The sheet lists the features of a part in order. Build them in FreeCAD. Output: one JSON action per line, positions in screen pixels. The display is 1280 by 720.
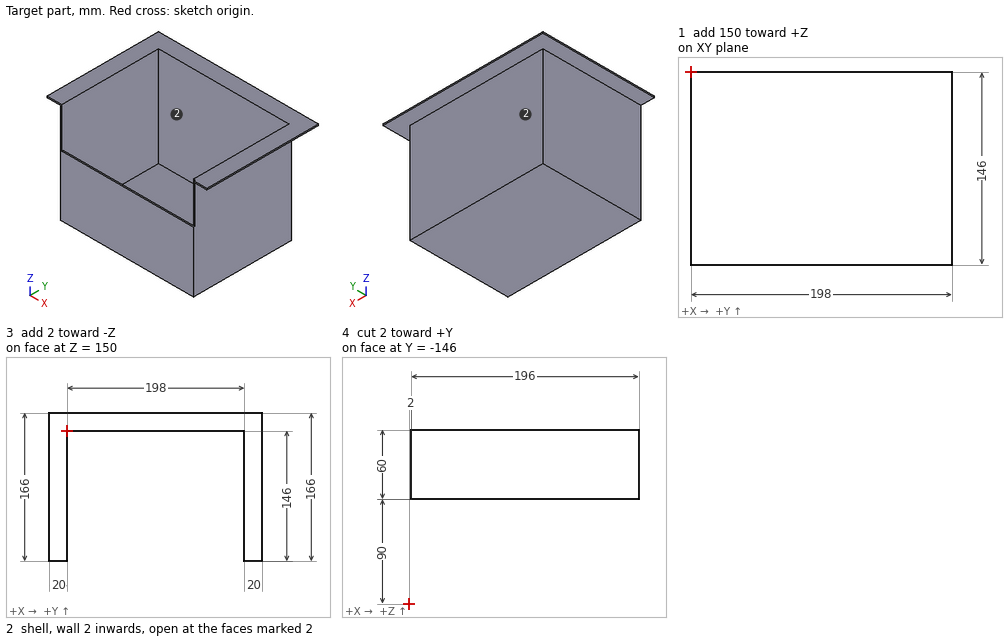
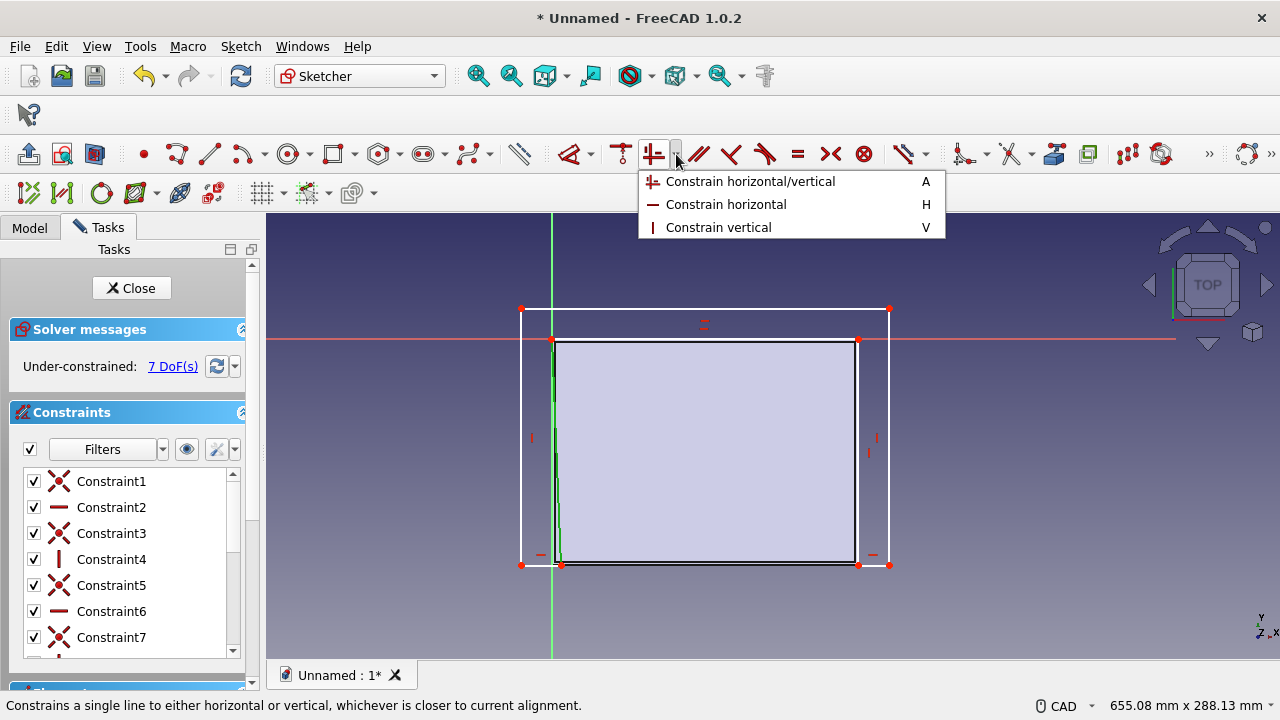
{"action": "left_click", "coordinate": [792, 228]}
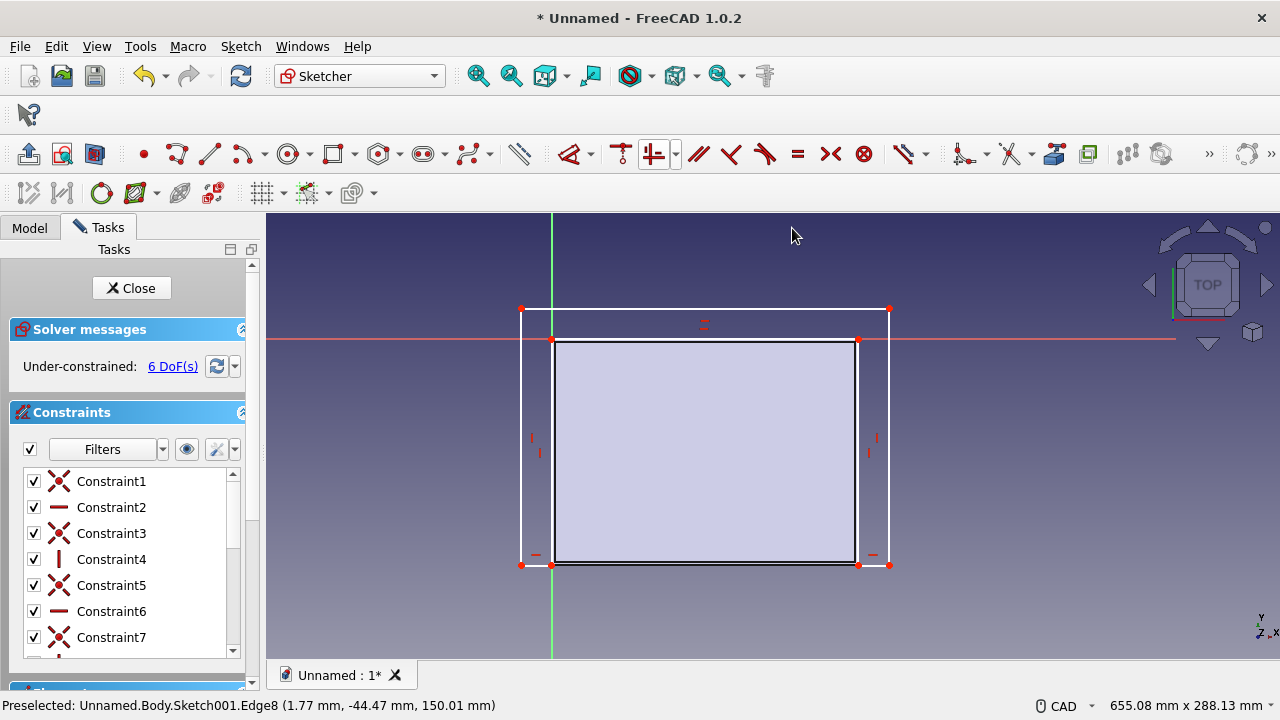
{"action": "left_click", "coordinate": [568, 154]}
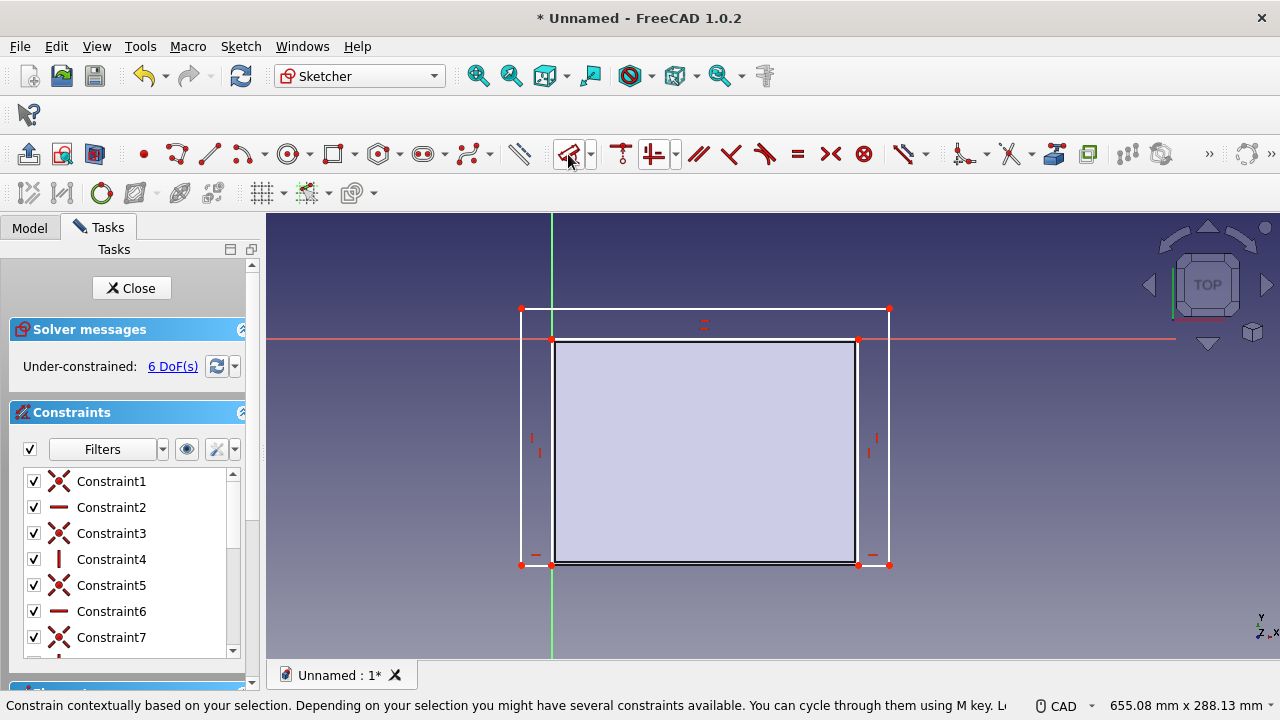
{"action": "scroll", "coordinate": [867, 566], "scroll_direction": "up", "scroll_amount": 2}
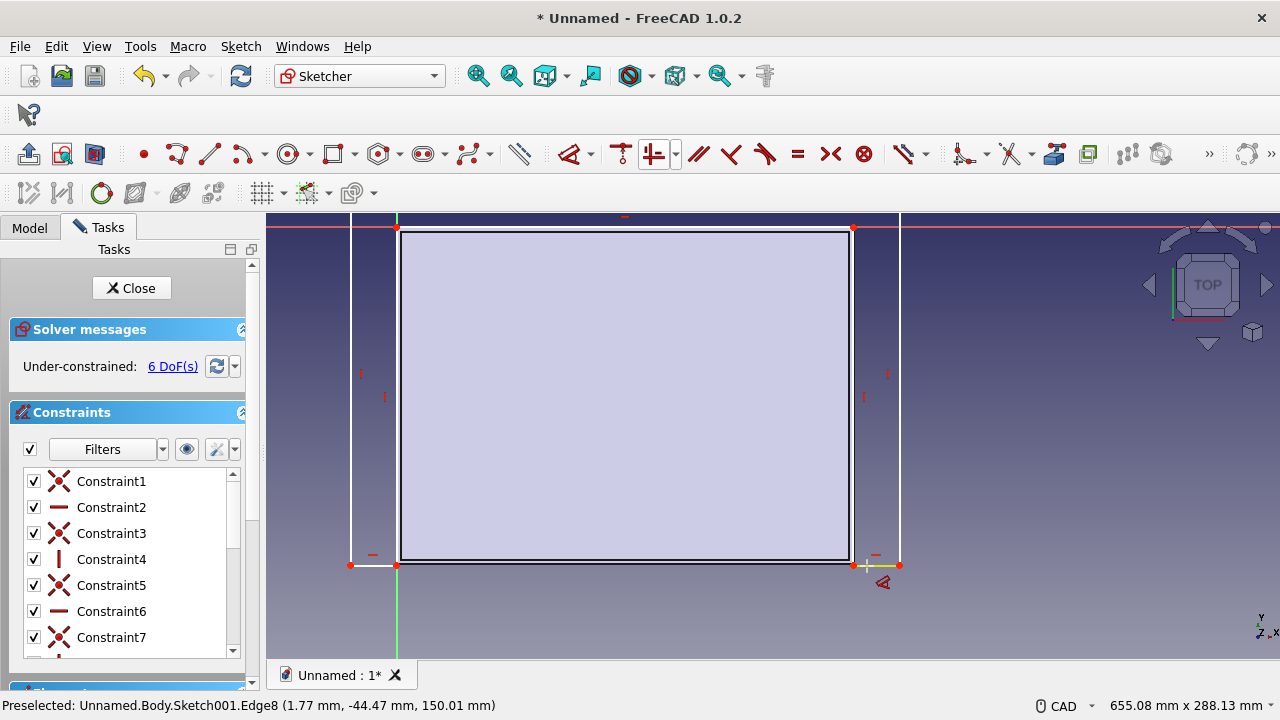
{"action": "left_click", "coordinate": [867, 566]}
{"action": "left_click", "coordinate": [876, 600]}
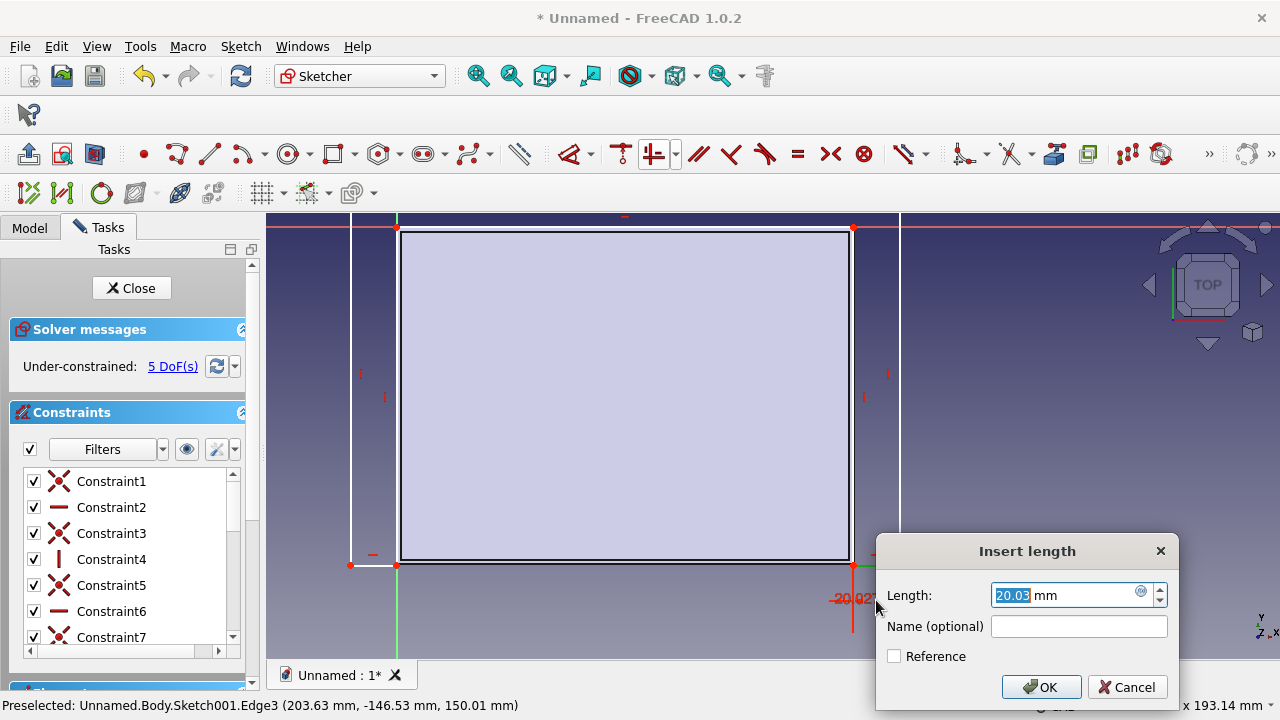
{"action": "type", "text": "20"}
{"action": "key", "text": "Return"}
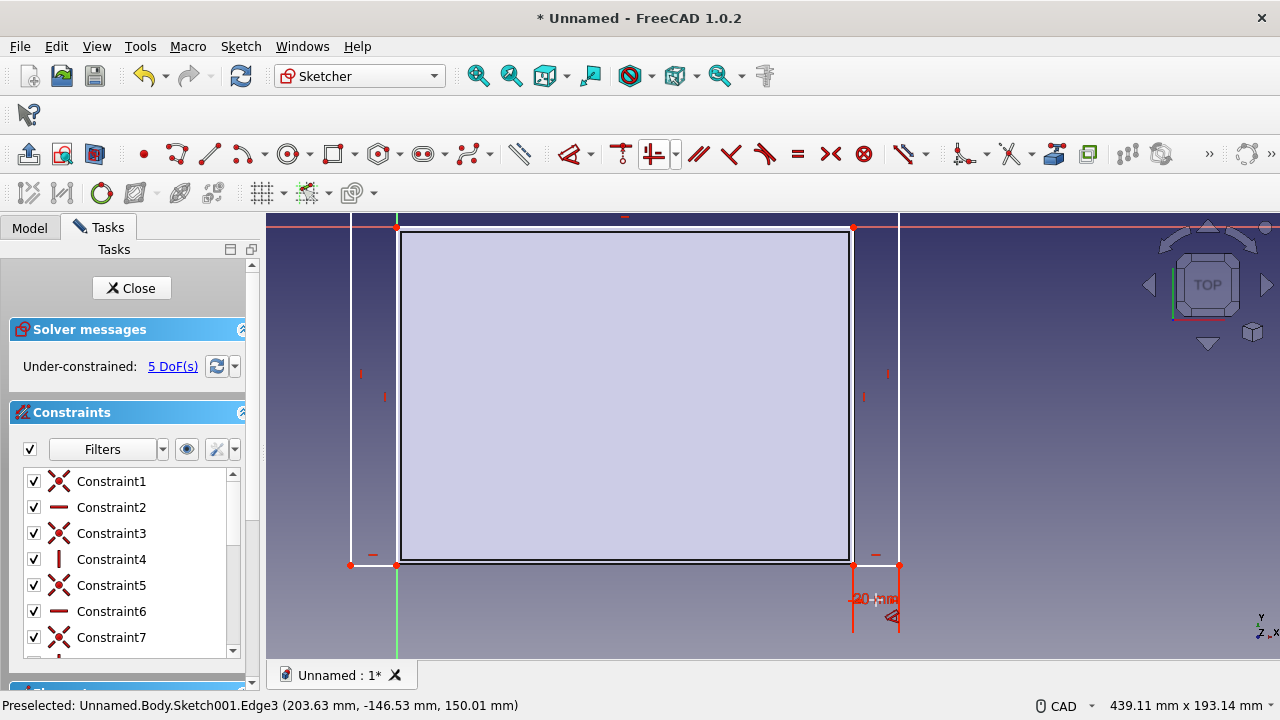
{"action": "left_click", "coordinate": [364, 566]}
{"action": "left_click", "coordinate": [374, 600]}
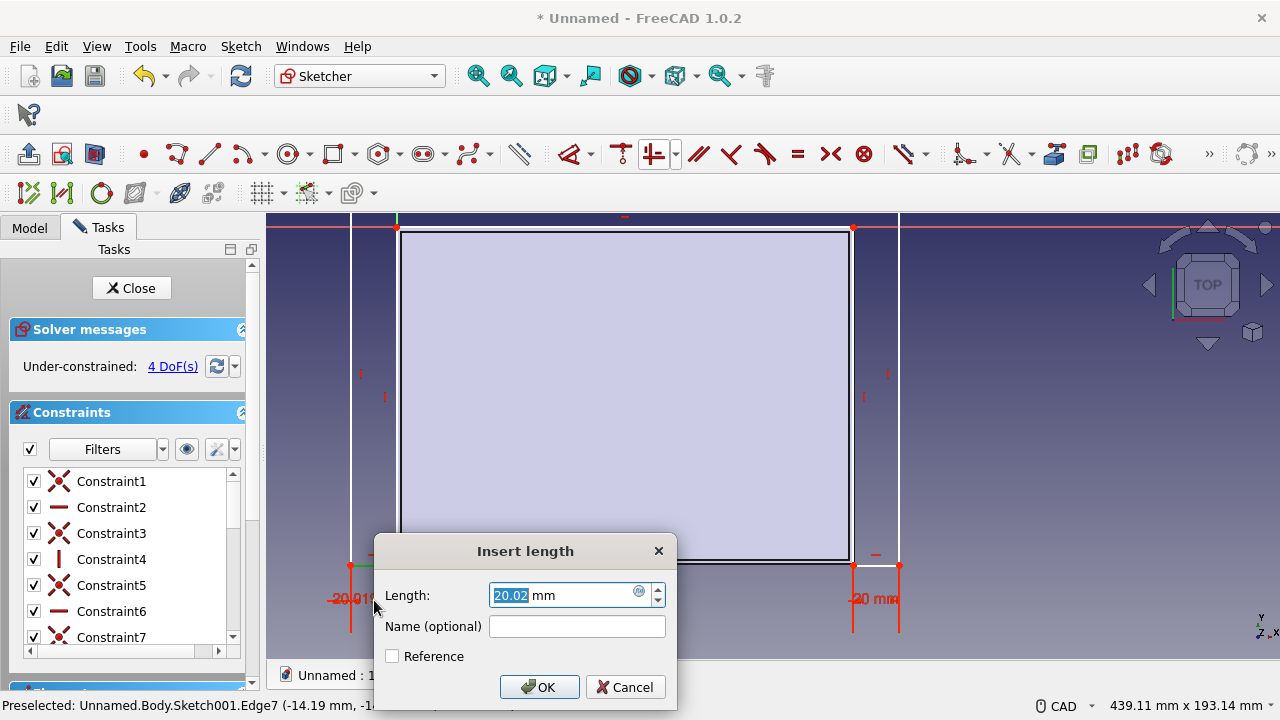
{"action": "type", "text": "20"}
{"action": "key", "text": "Return"}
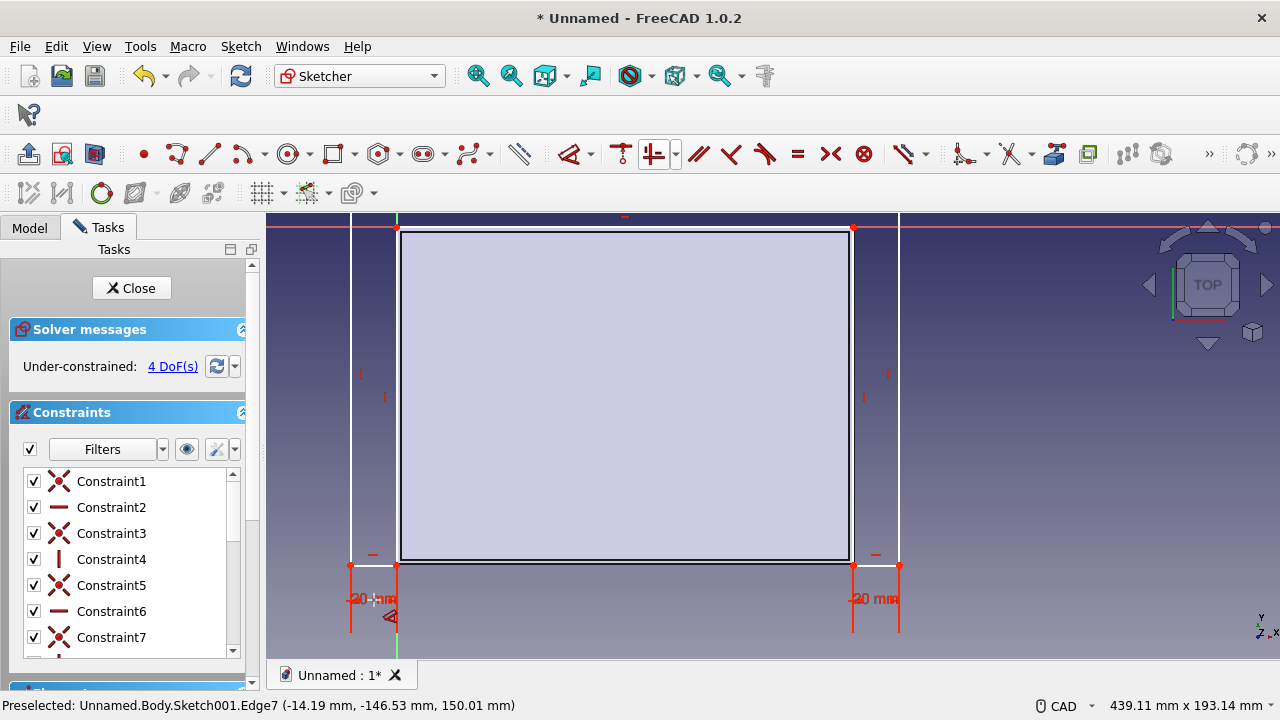
{"action": "scroll", "coordinate": [865, 565], "scroll_direction": "down", "scroll_amount": 2}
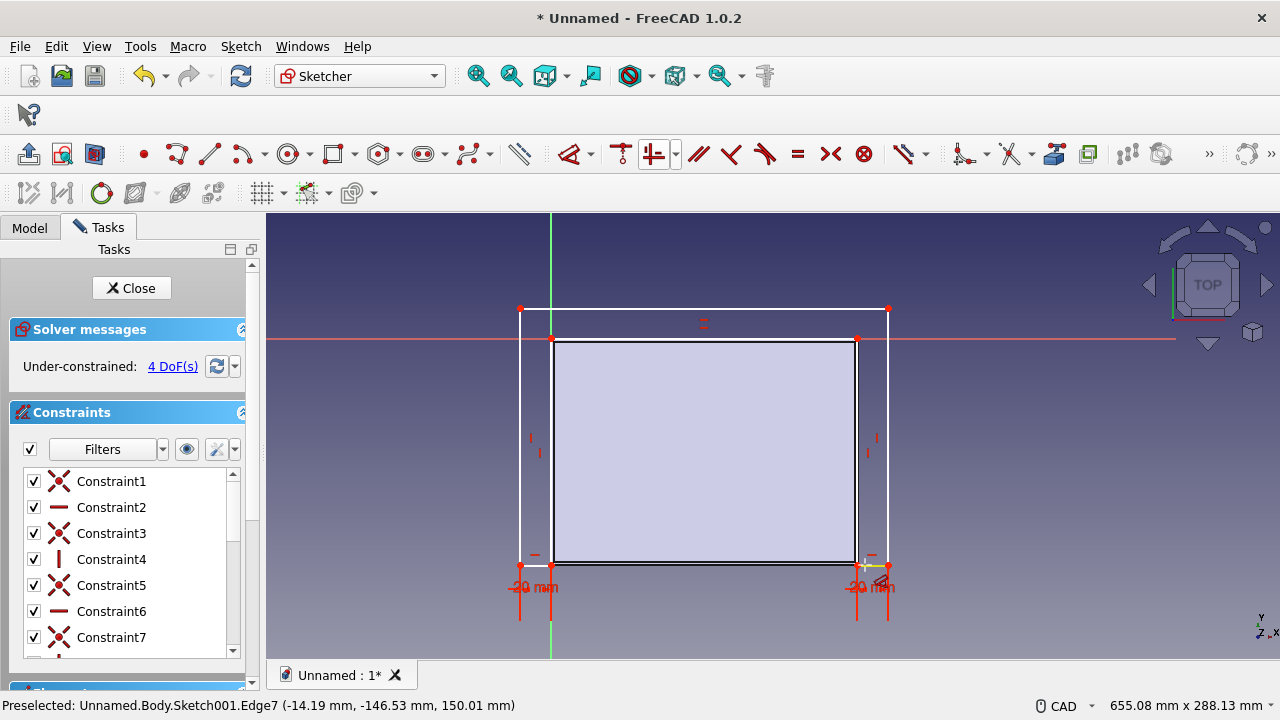
{"action": "left_click", "coordinate": [643, 339]}
{"action": "left_click", "coordinate": [704, 373]}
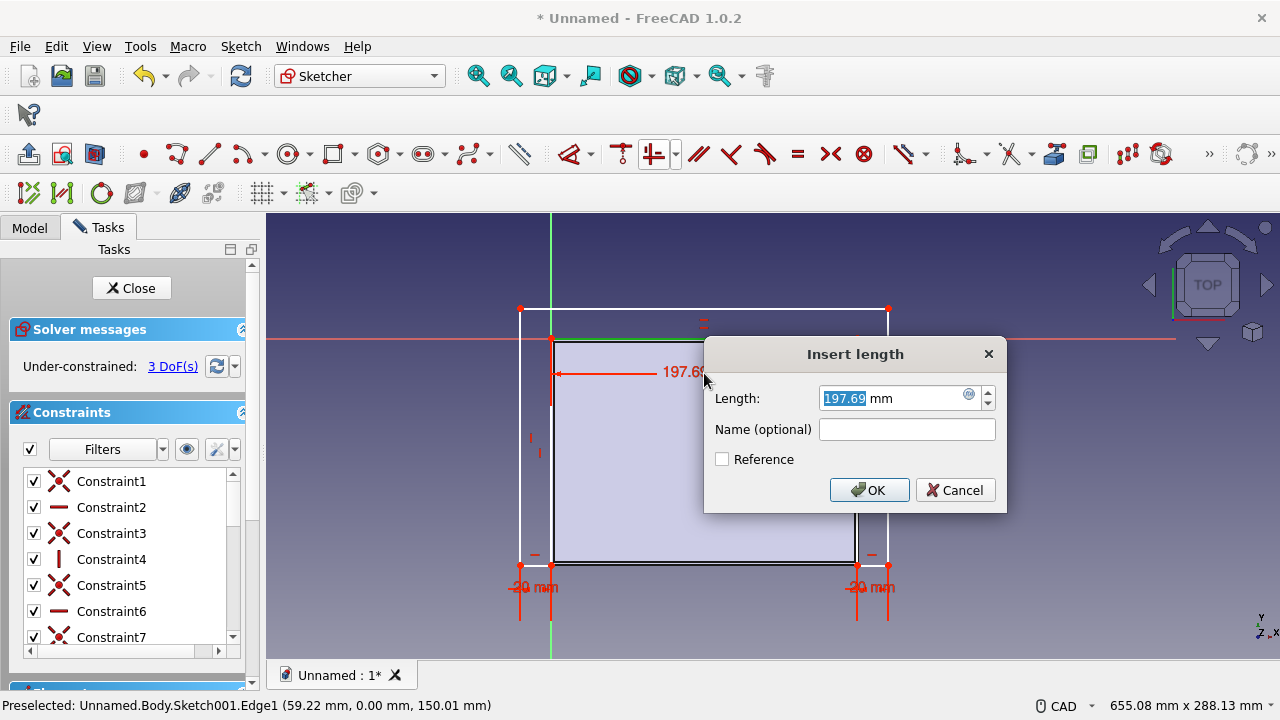
{"action": "type", "text": "198"}
{"action": "key", "text": "Return"}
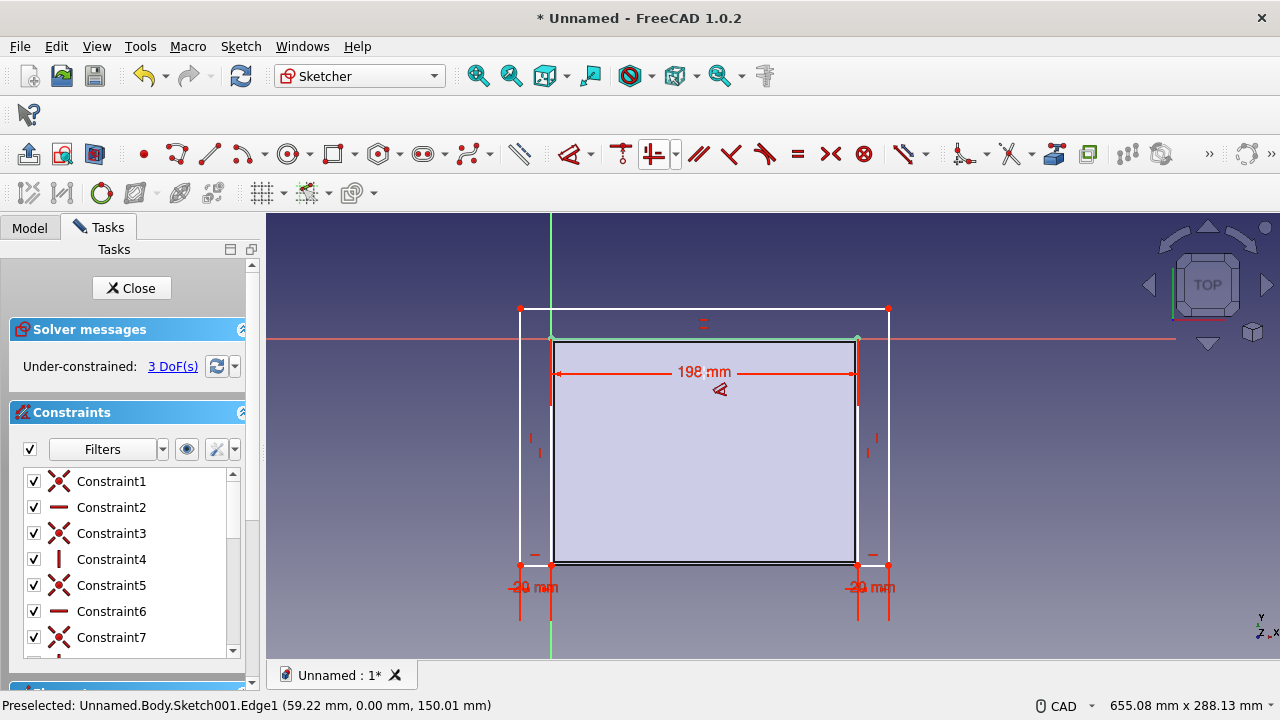
{"action": "left_click", "coordinate": [858, 407]}
{"action": "left_click", "coordinate": [824, 452]}